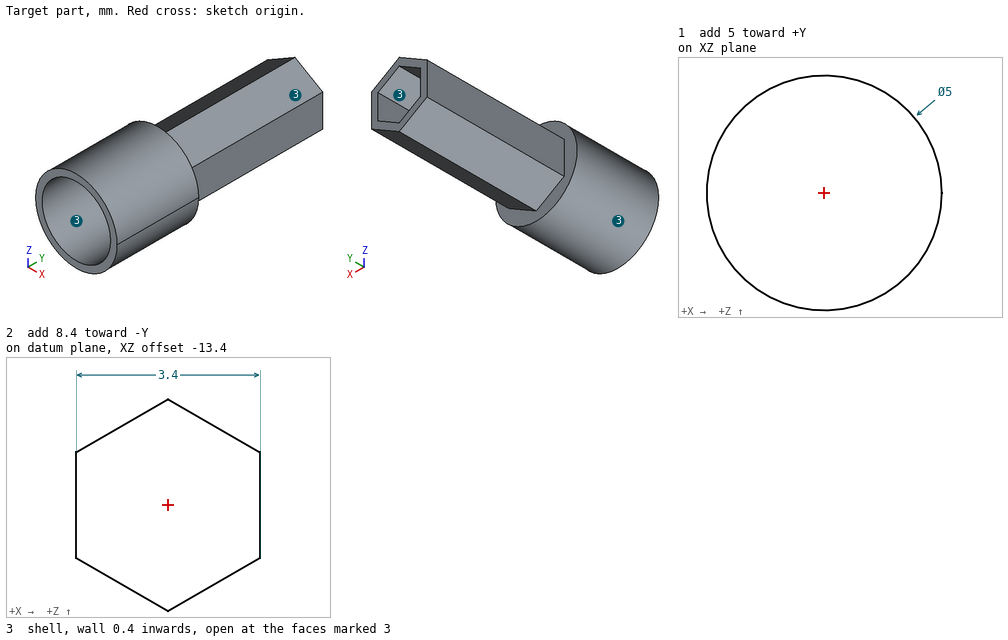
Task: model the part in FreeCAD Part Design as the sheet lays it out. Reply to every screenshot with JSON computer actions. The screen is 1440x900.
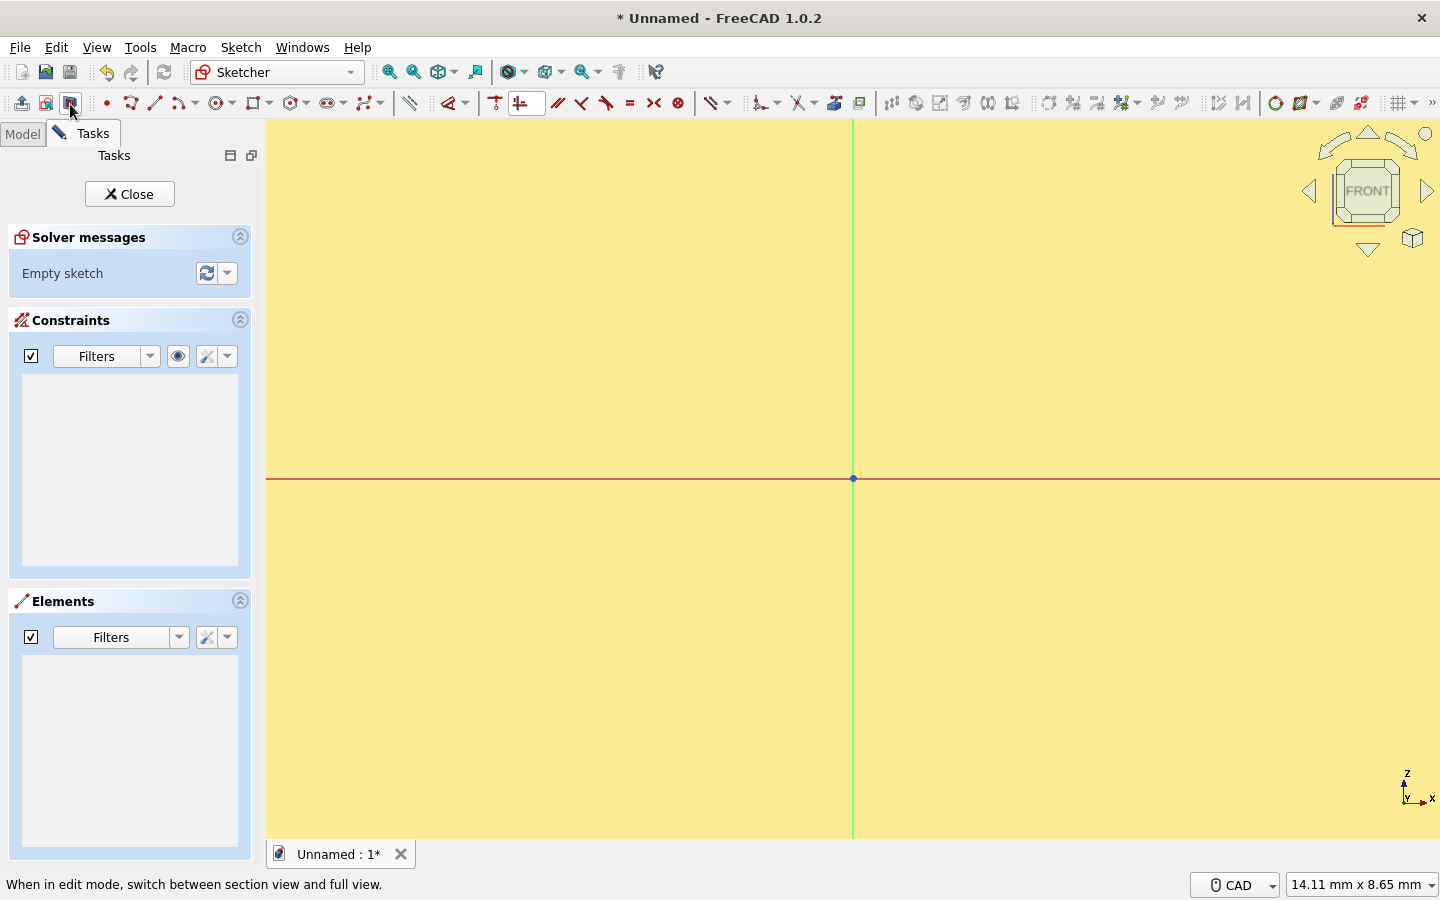
{"action": "scroll", "coordinate": [992, 479], "scroll_direction": "up", "scroll_amount": 2}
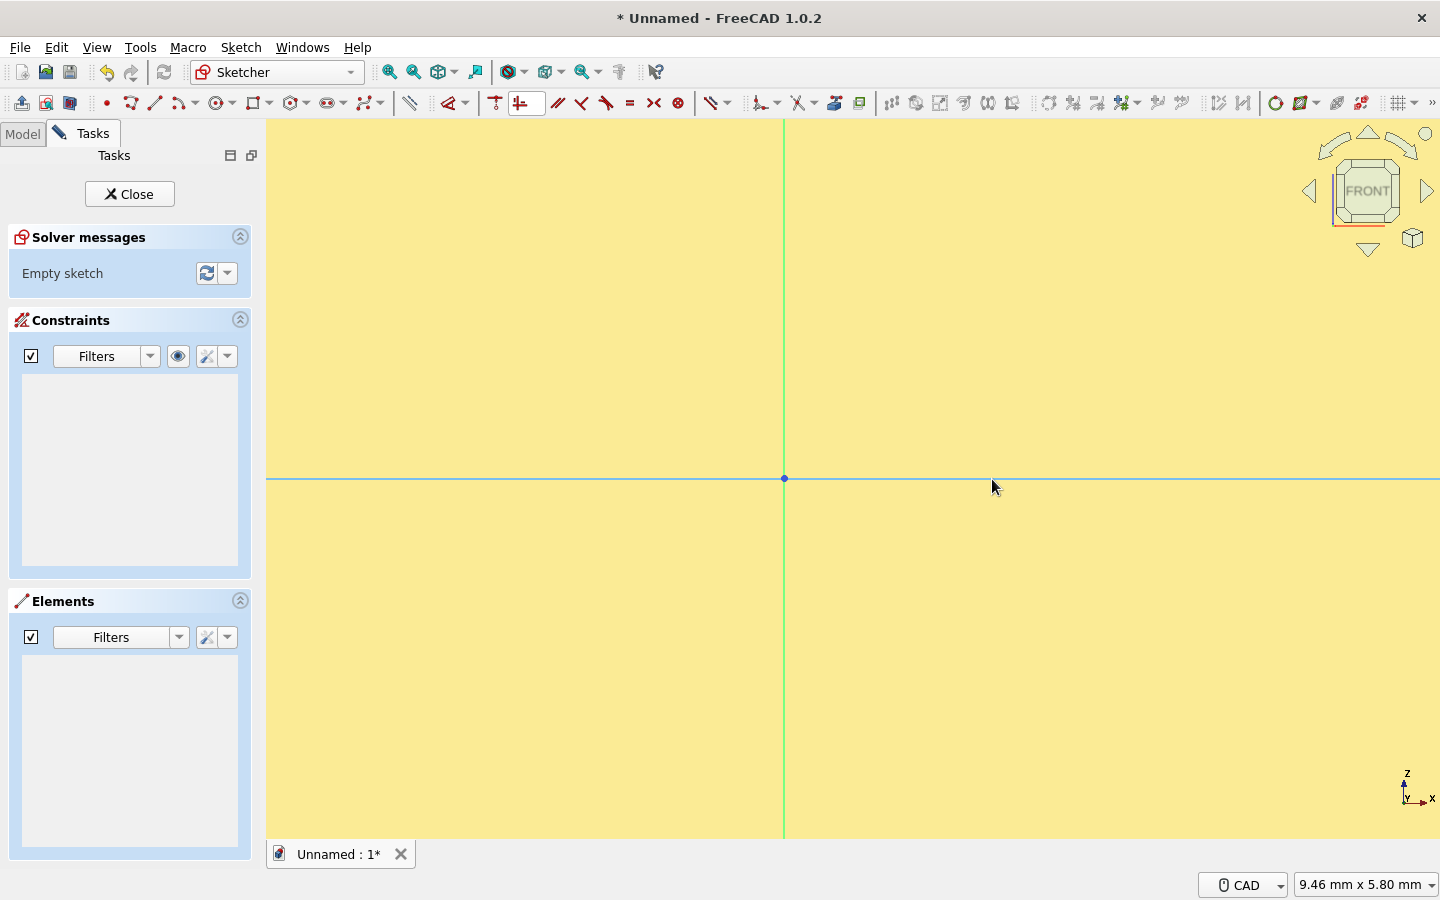
{"action": "left_click", "coordinate": [290, 104]}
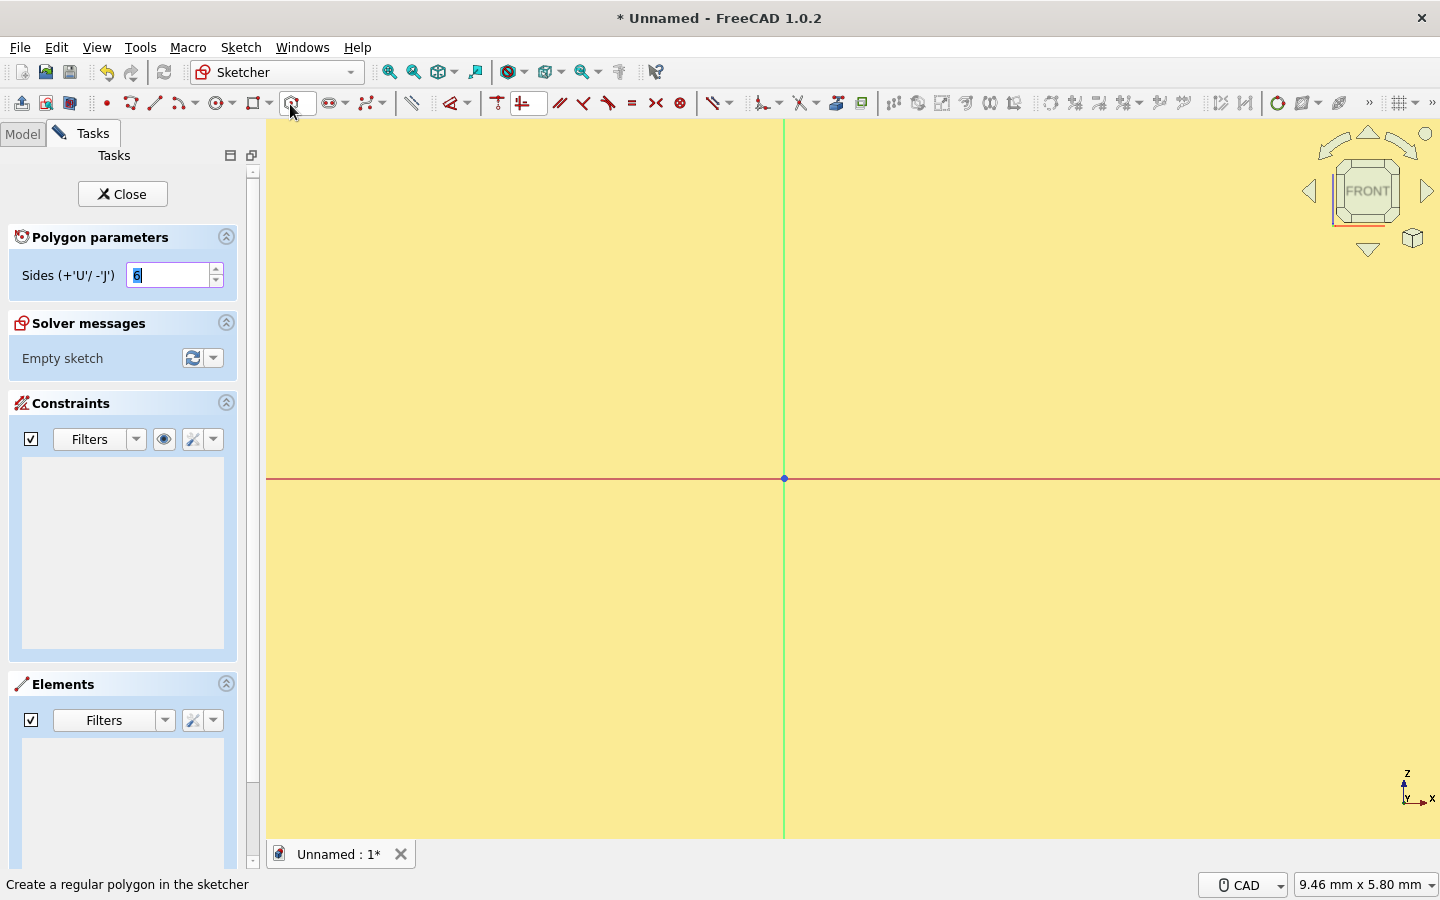
{"action": "left_click", "coordinate": [784, 479]}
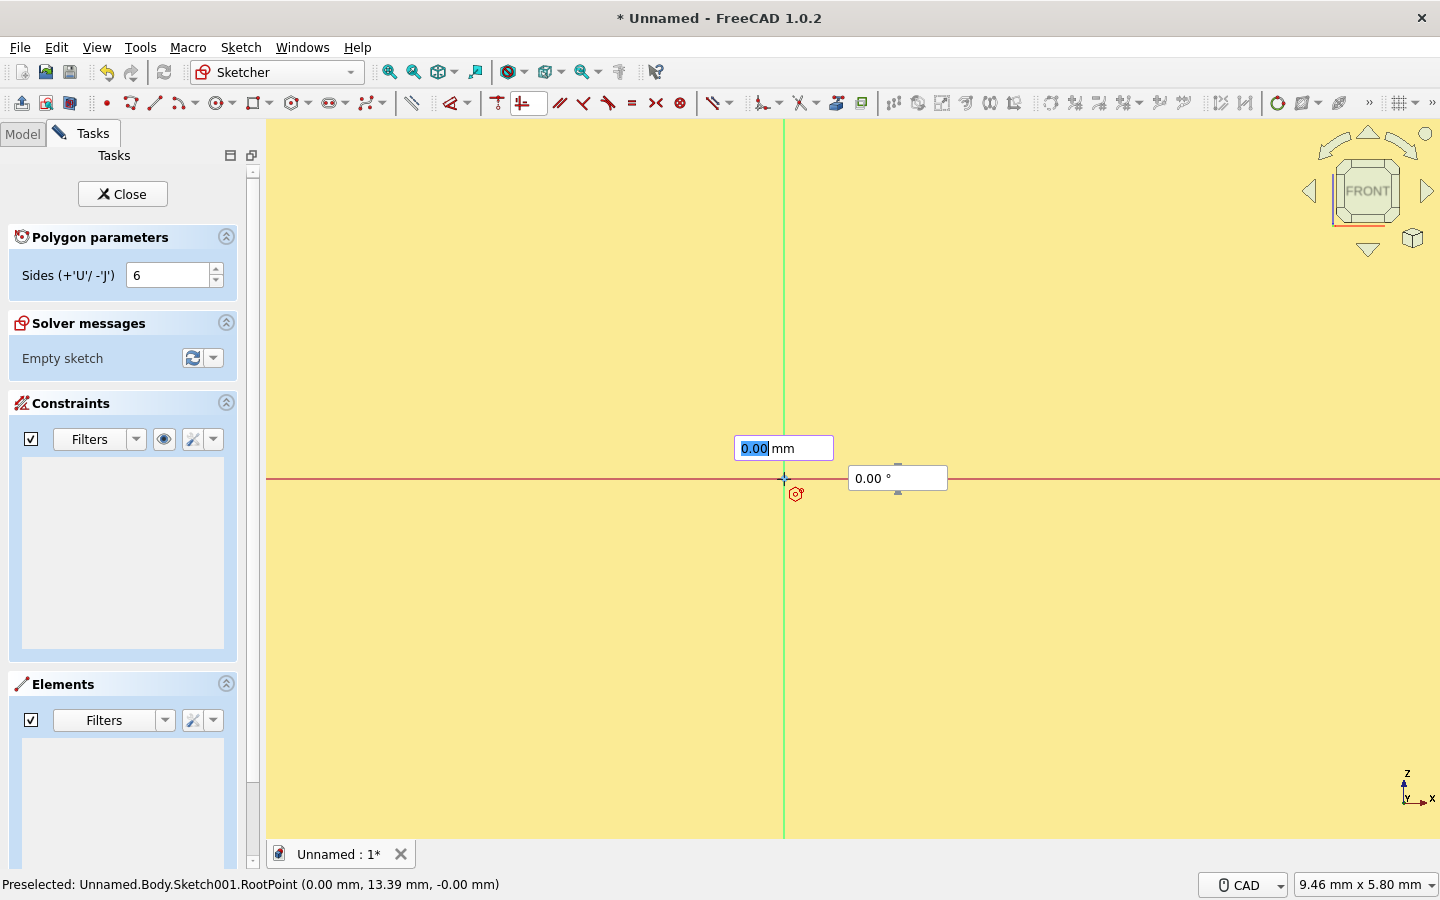
{"action": "left_click", "coordinate": [784, 722]}
{"action": "key", "text": "Escape"}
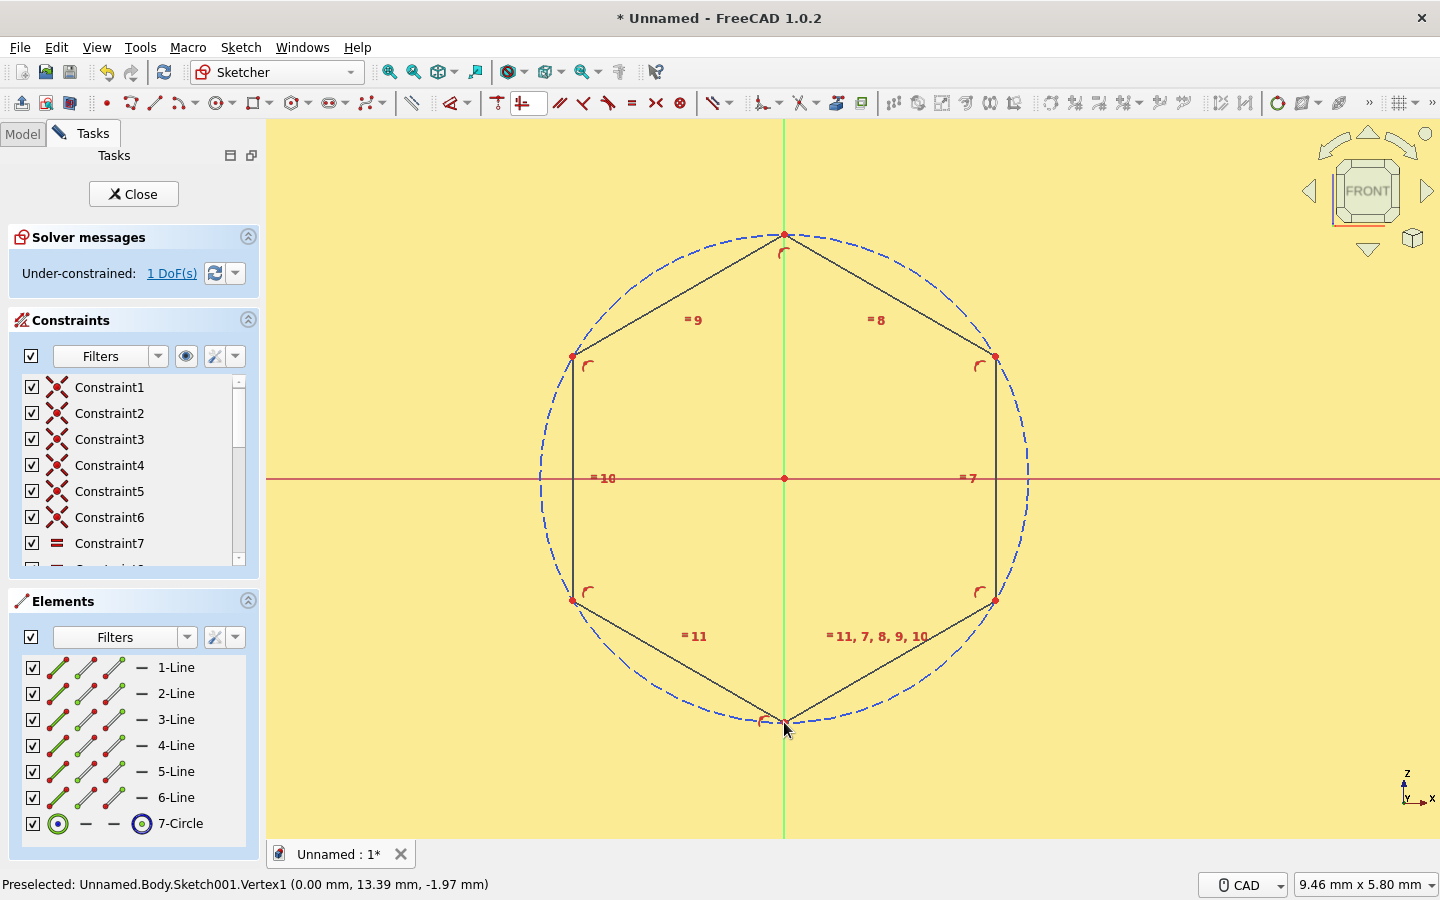
{"action": "left_click", "coordinate": [573, 357]}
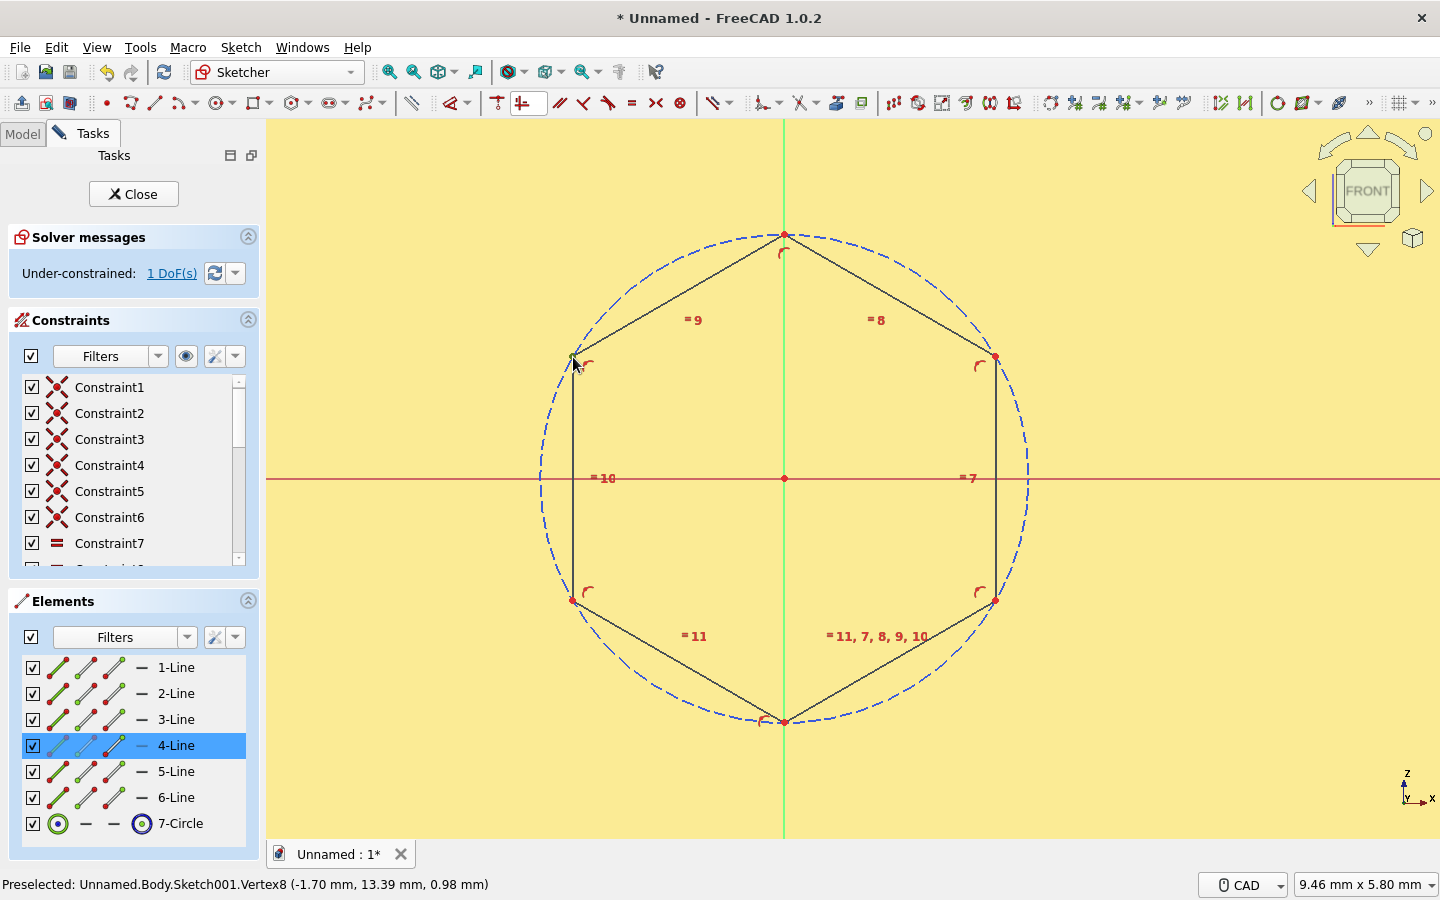
{"action": "left_click", "coordinate": [996, 601]}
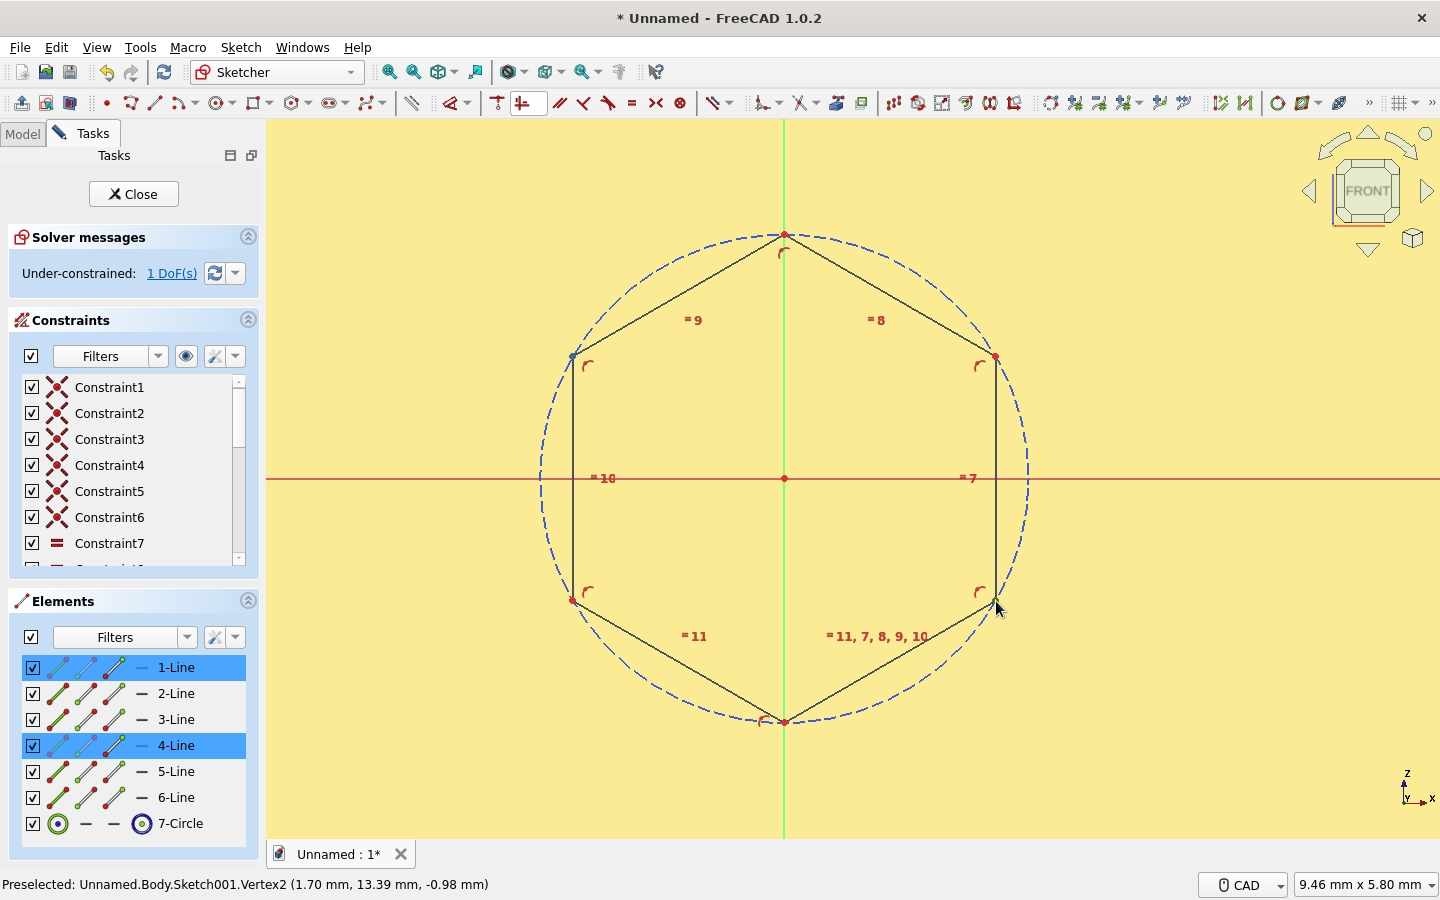
{"action": "left_click", "coordinate": [470, 104]}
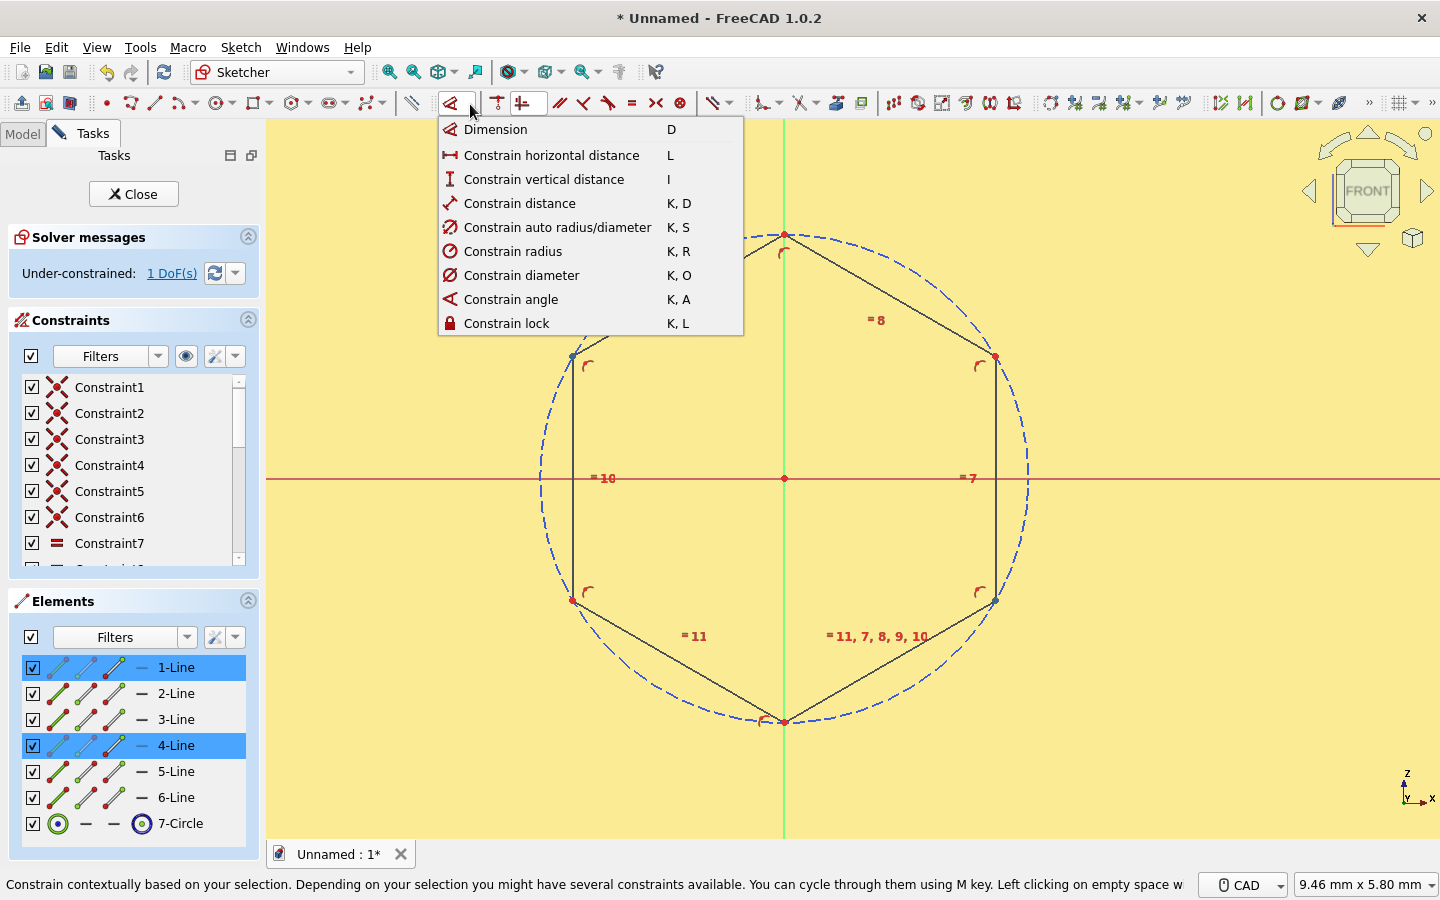
{"action": "left_click", "coordinate": [591, 155]}